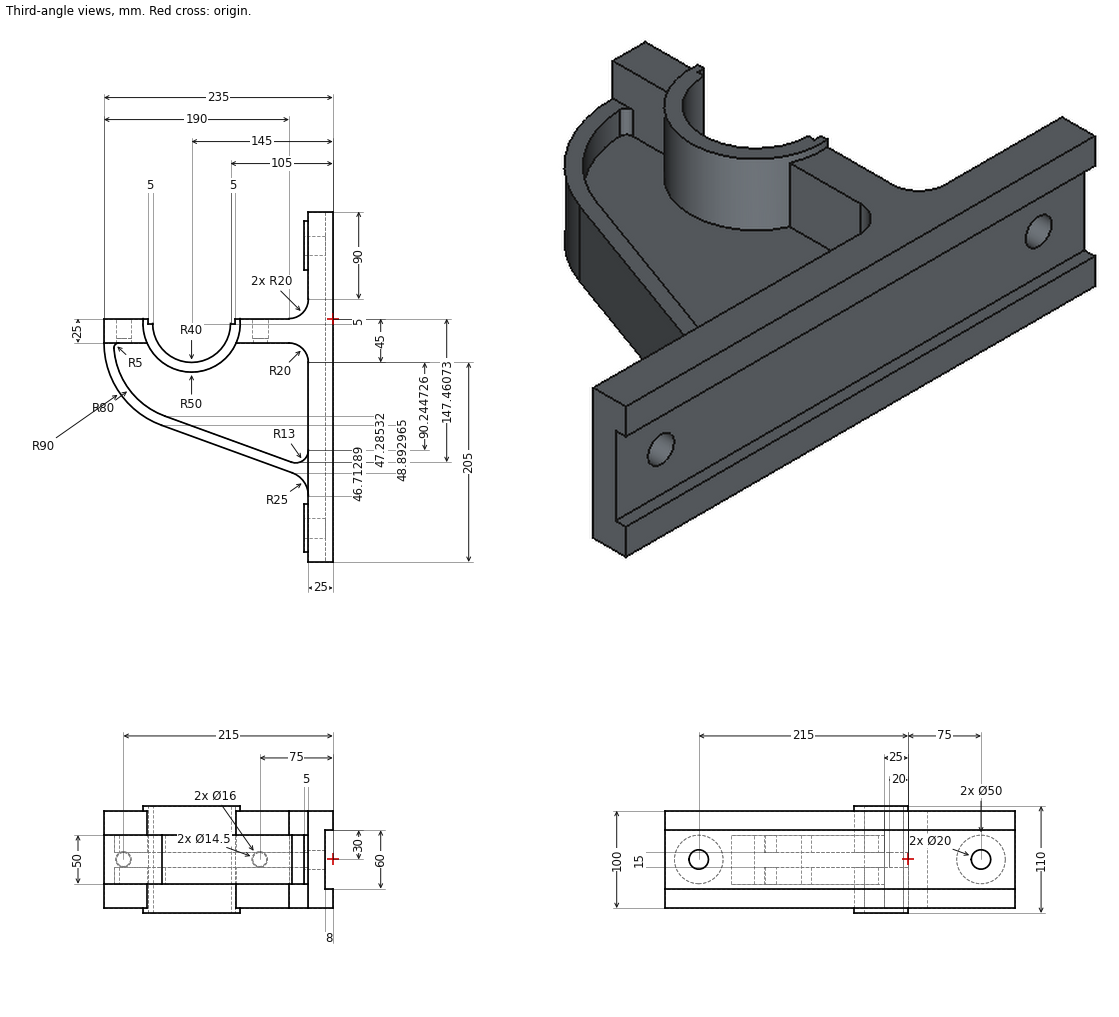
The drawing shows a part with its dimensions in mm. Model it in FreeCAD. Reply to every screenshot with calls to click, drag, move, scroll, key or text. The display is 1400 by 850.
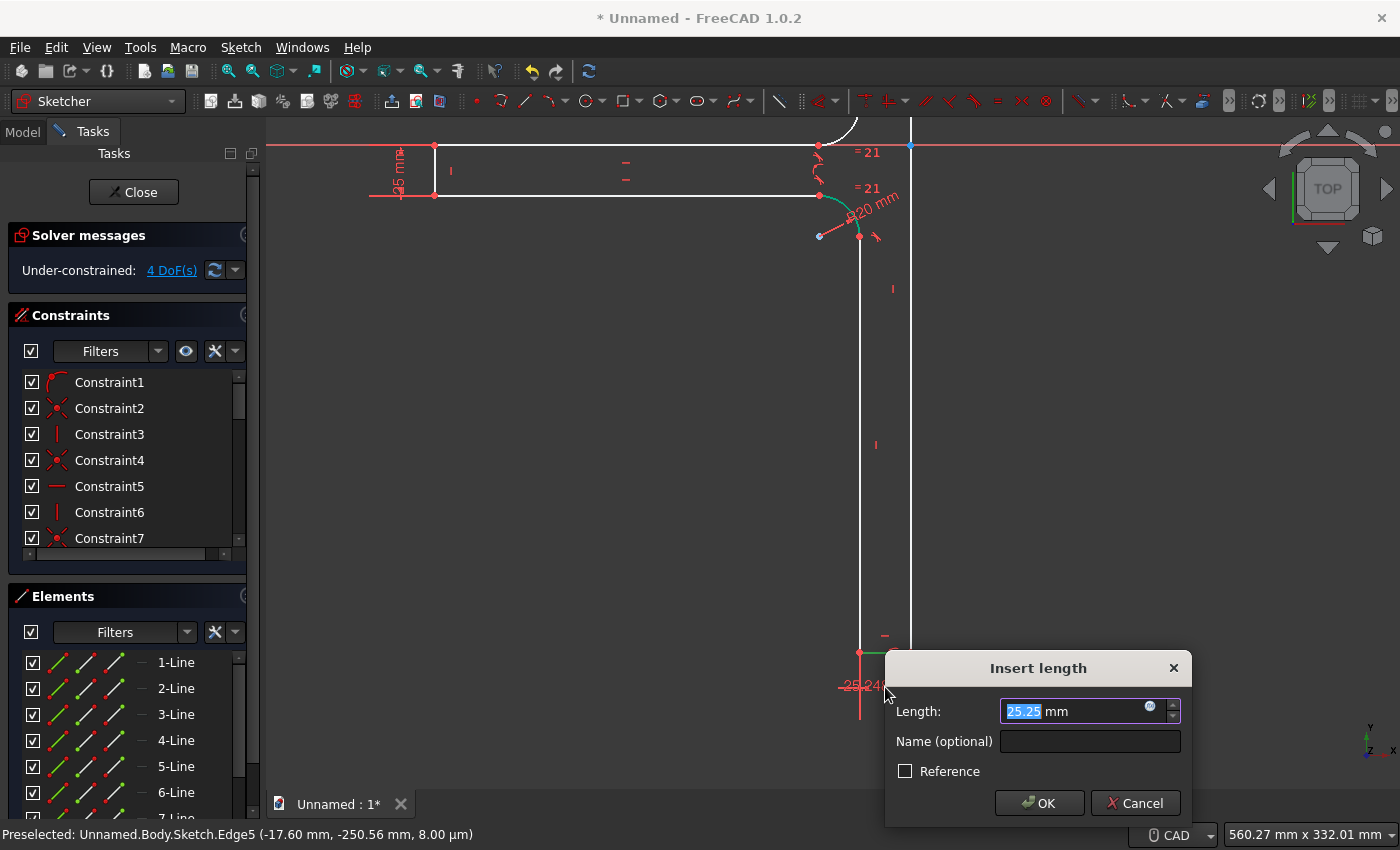
text(25)
key(Return)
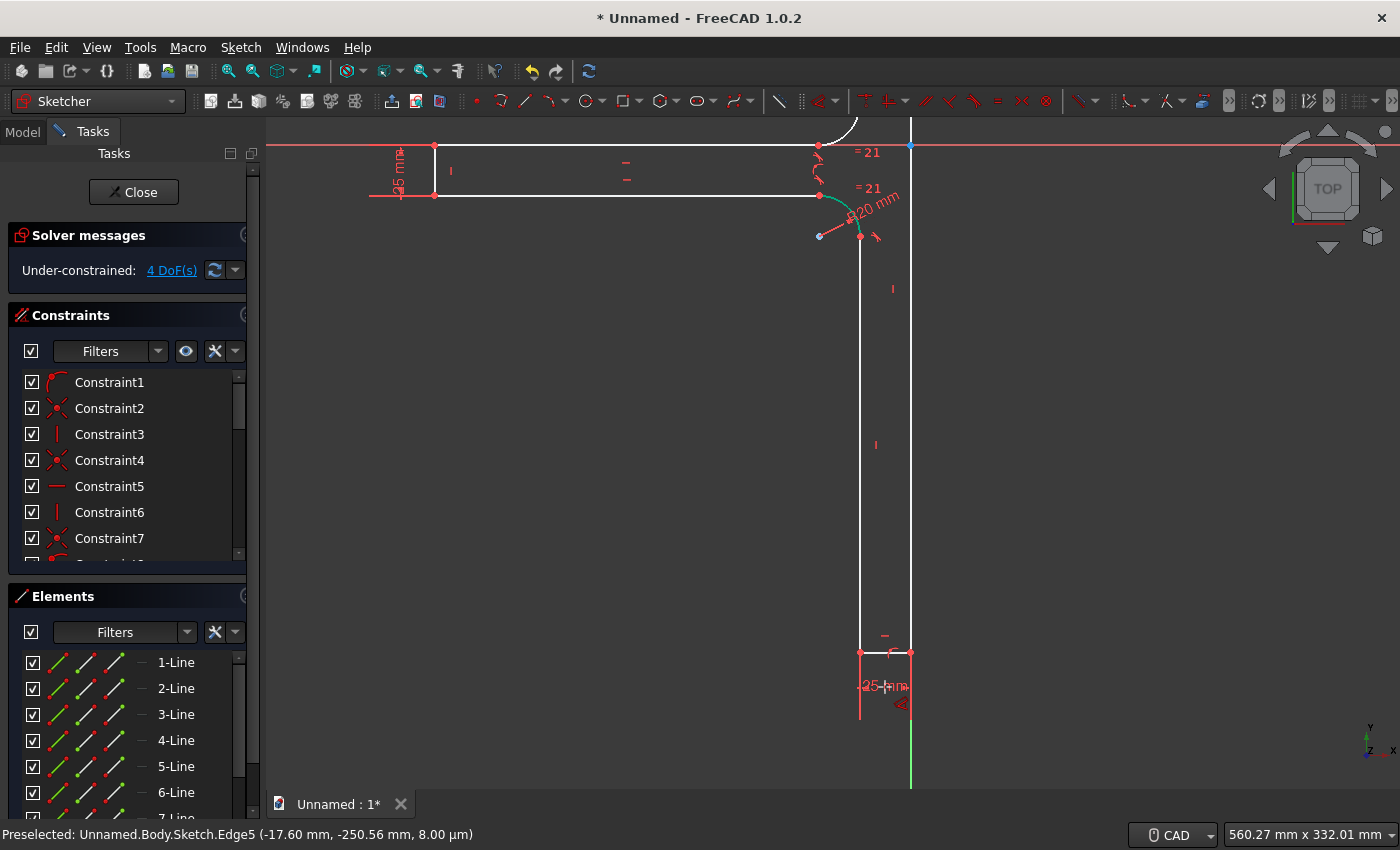
scroll(876, 655, down, 3)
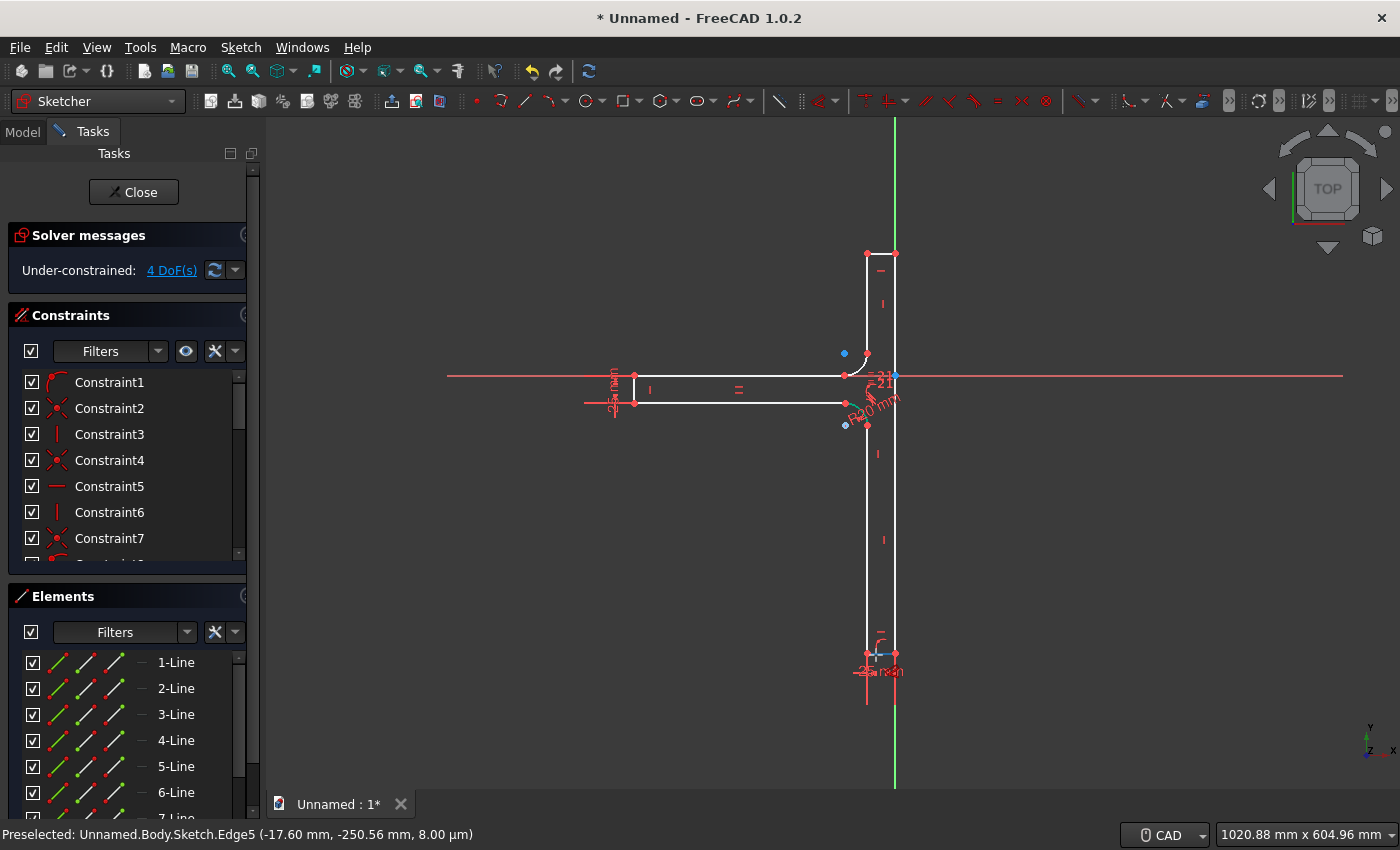
scroll(887, 254, up, 3)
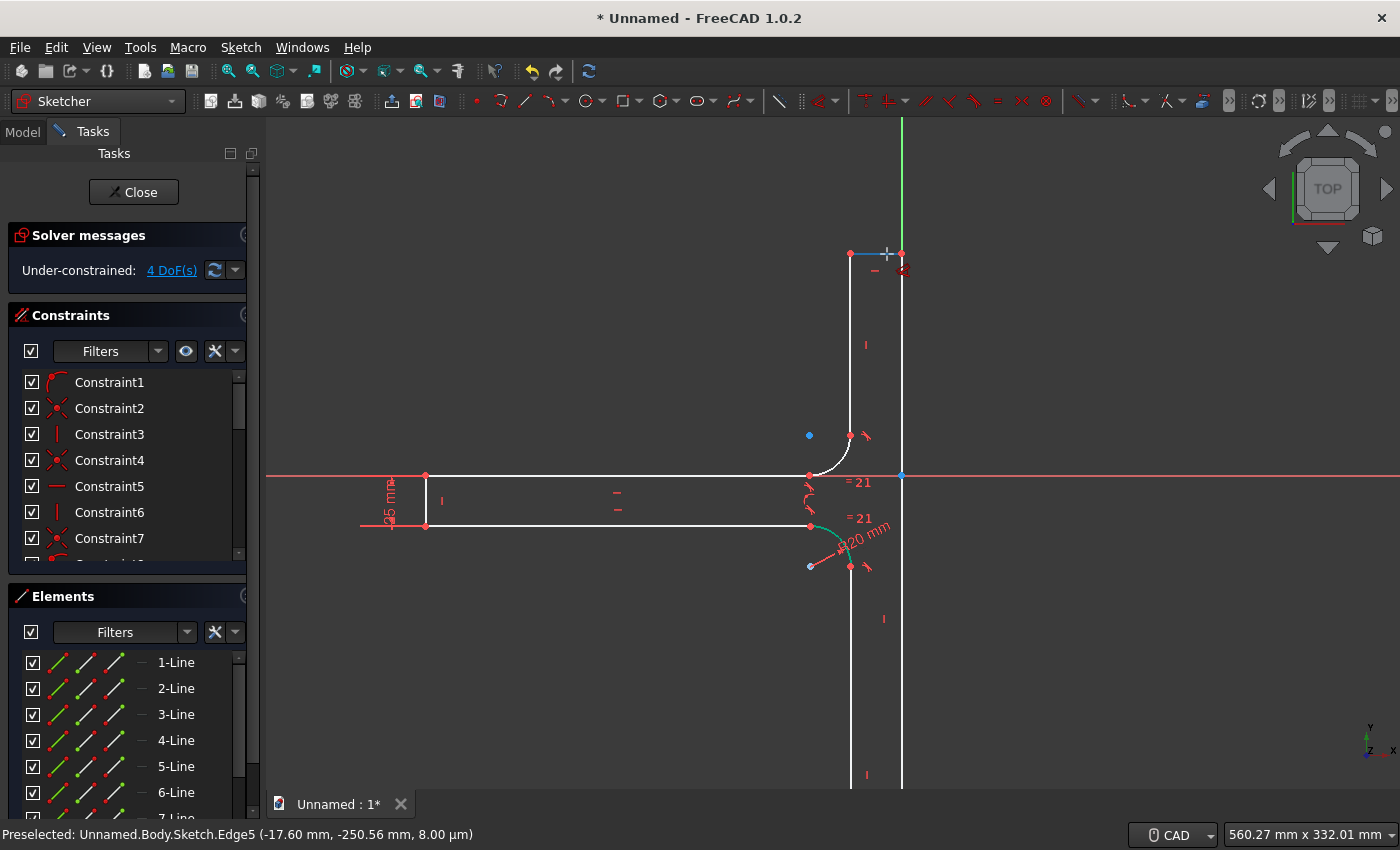
click(886, 254)
click(876, 220)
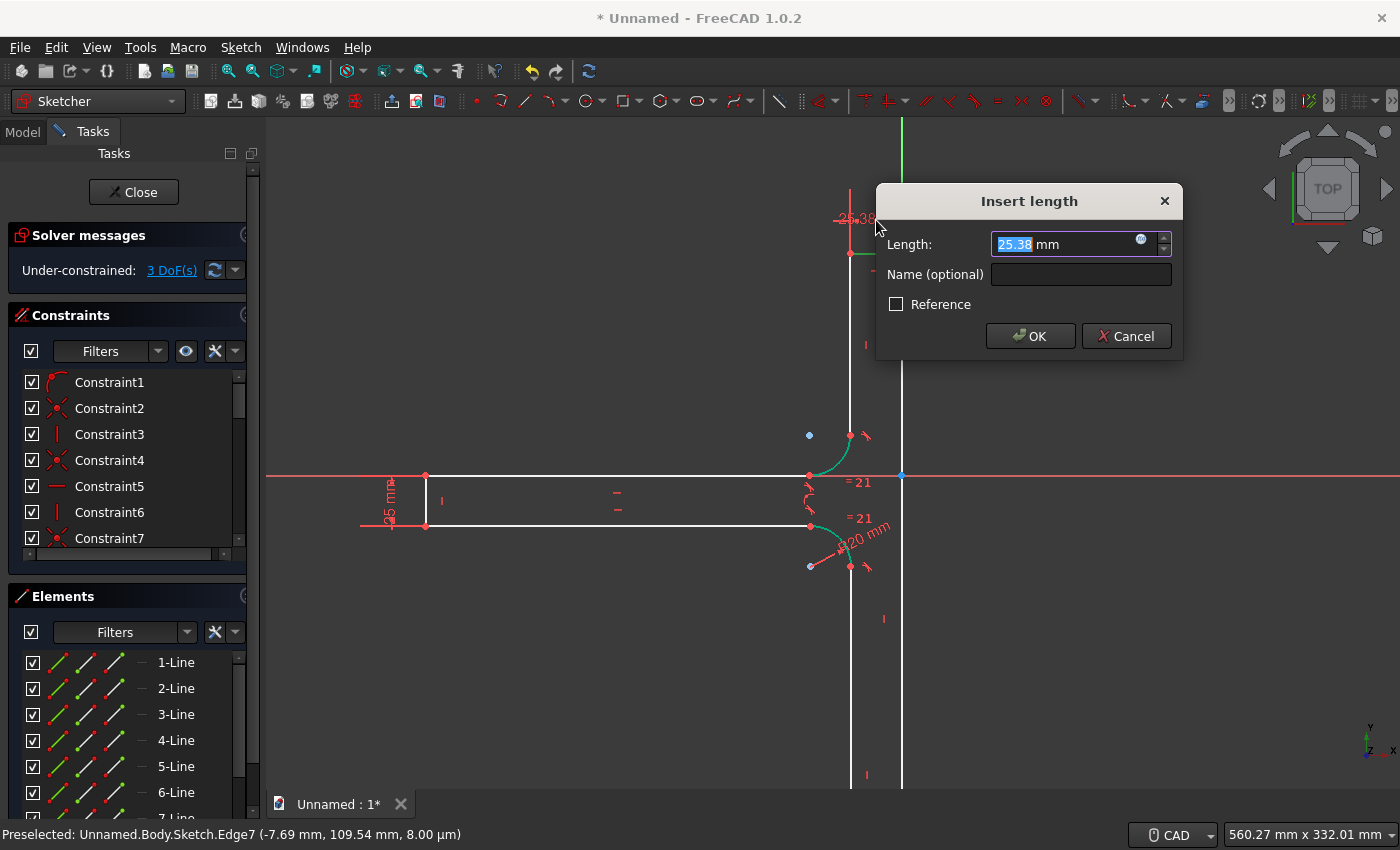
text(25)
key(Return)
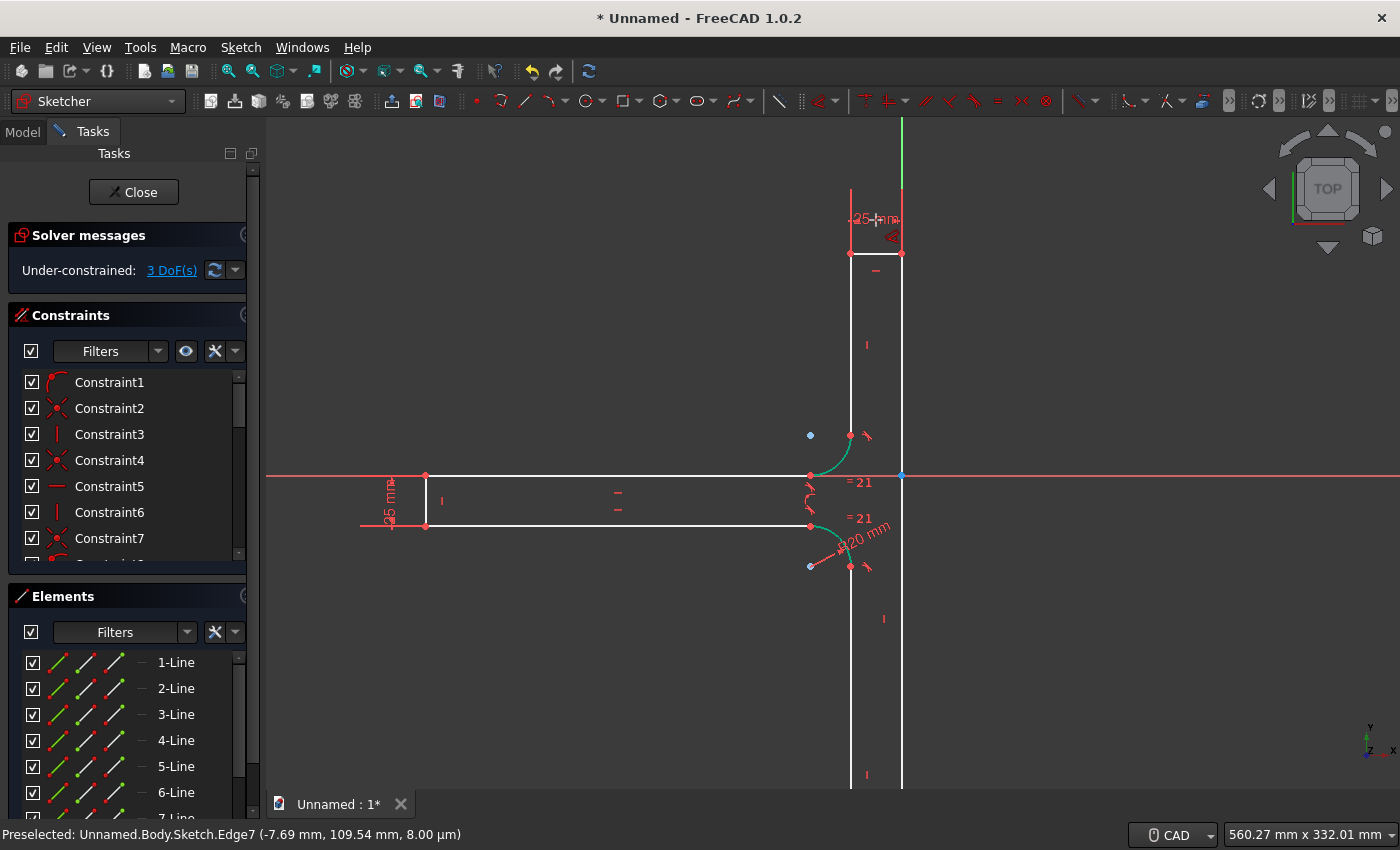
click(851, 308)
click(885, 344)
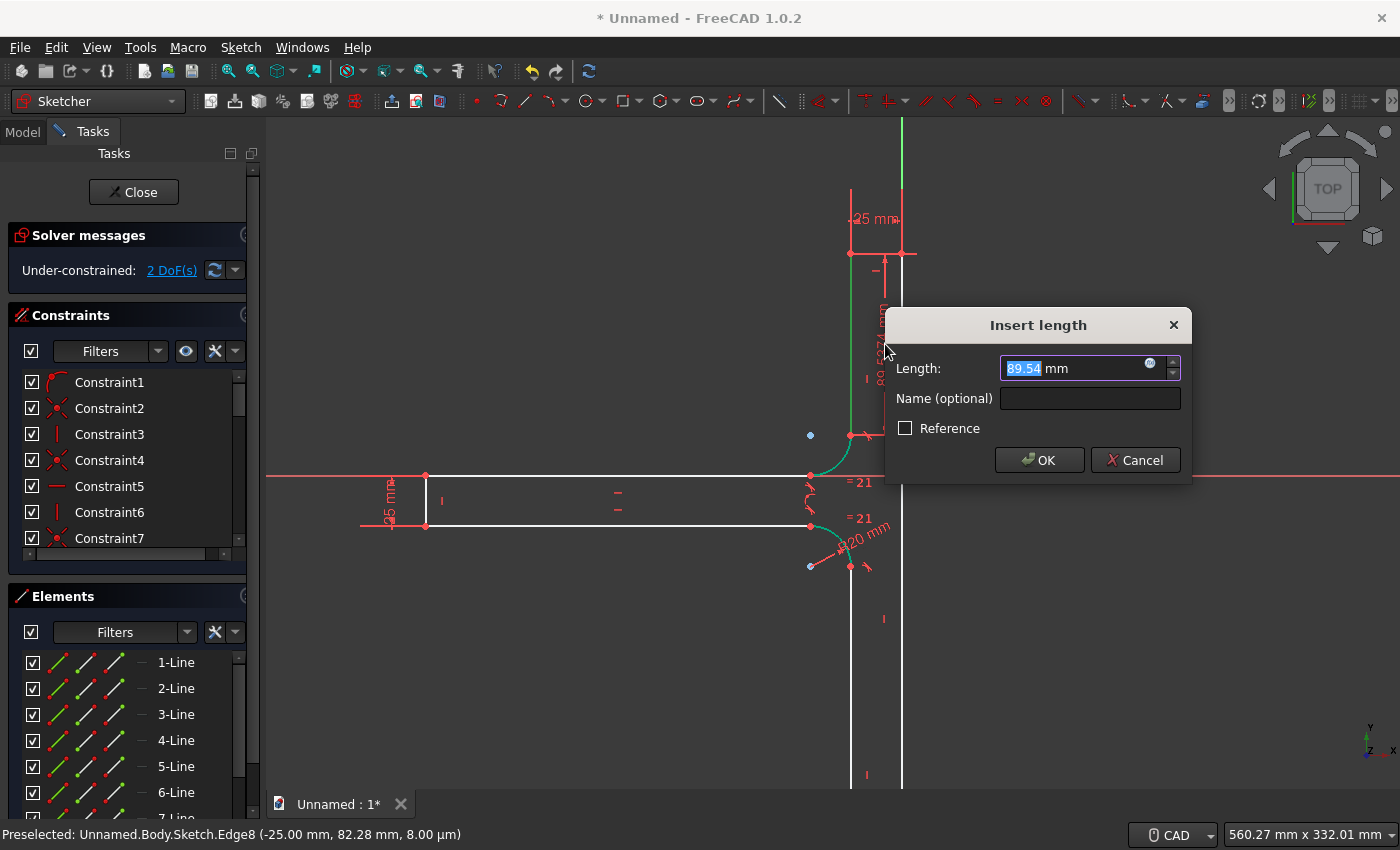
text(90)
key(Return)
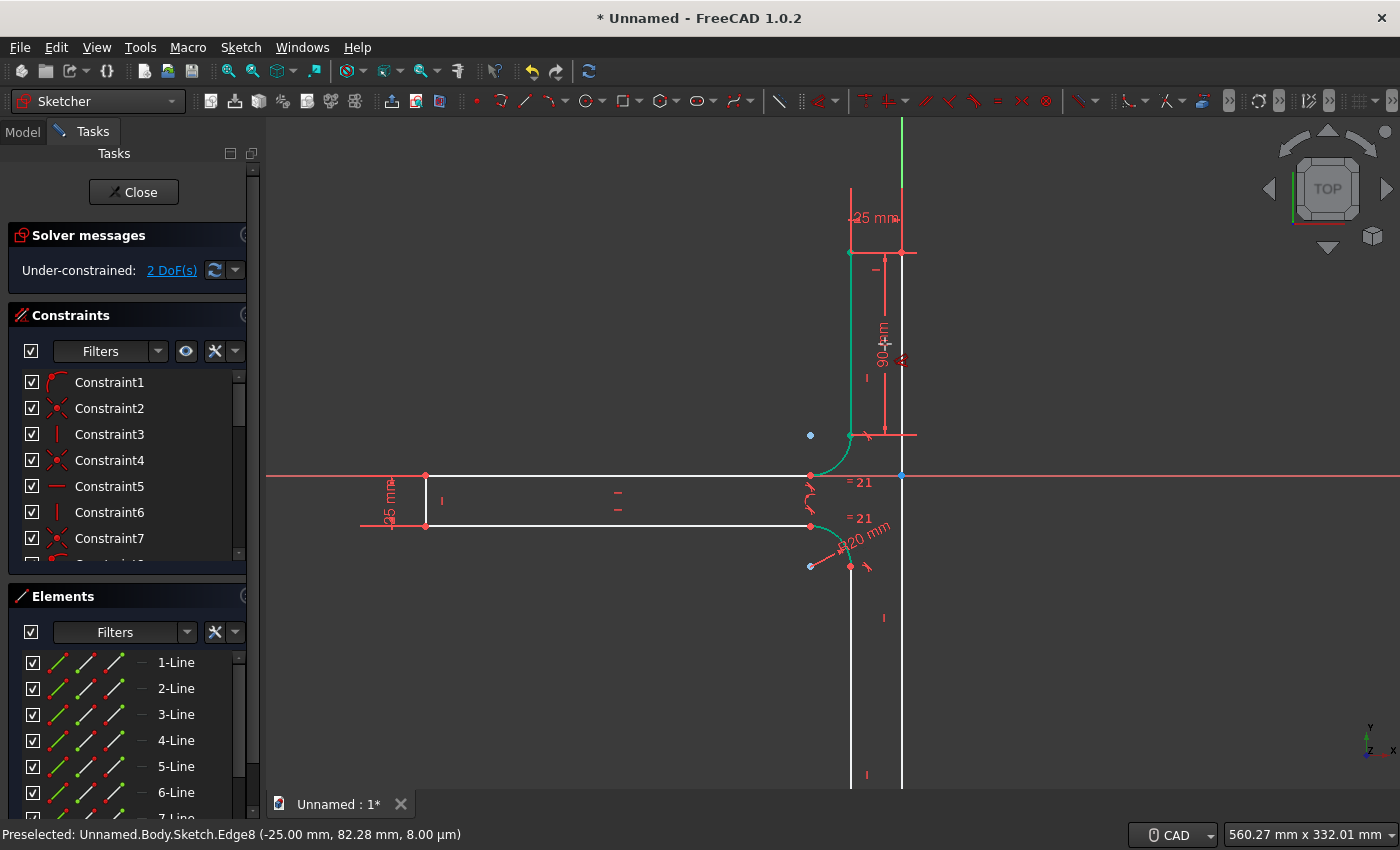
click(695, 476)
click(618, 442)